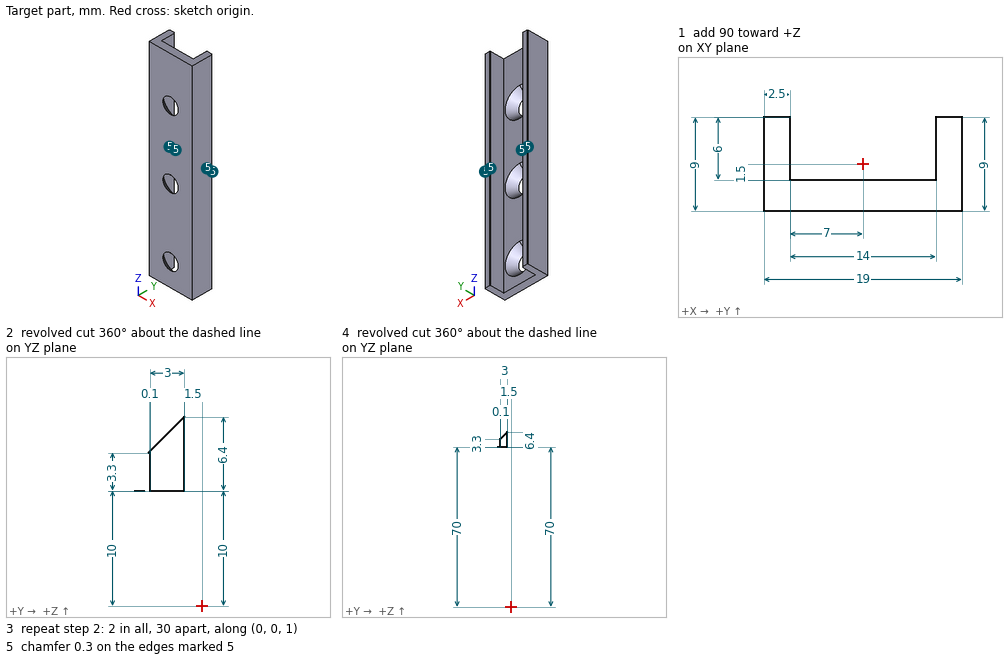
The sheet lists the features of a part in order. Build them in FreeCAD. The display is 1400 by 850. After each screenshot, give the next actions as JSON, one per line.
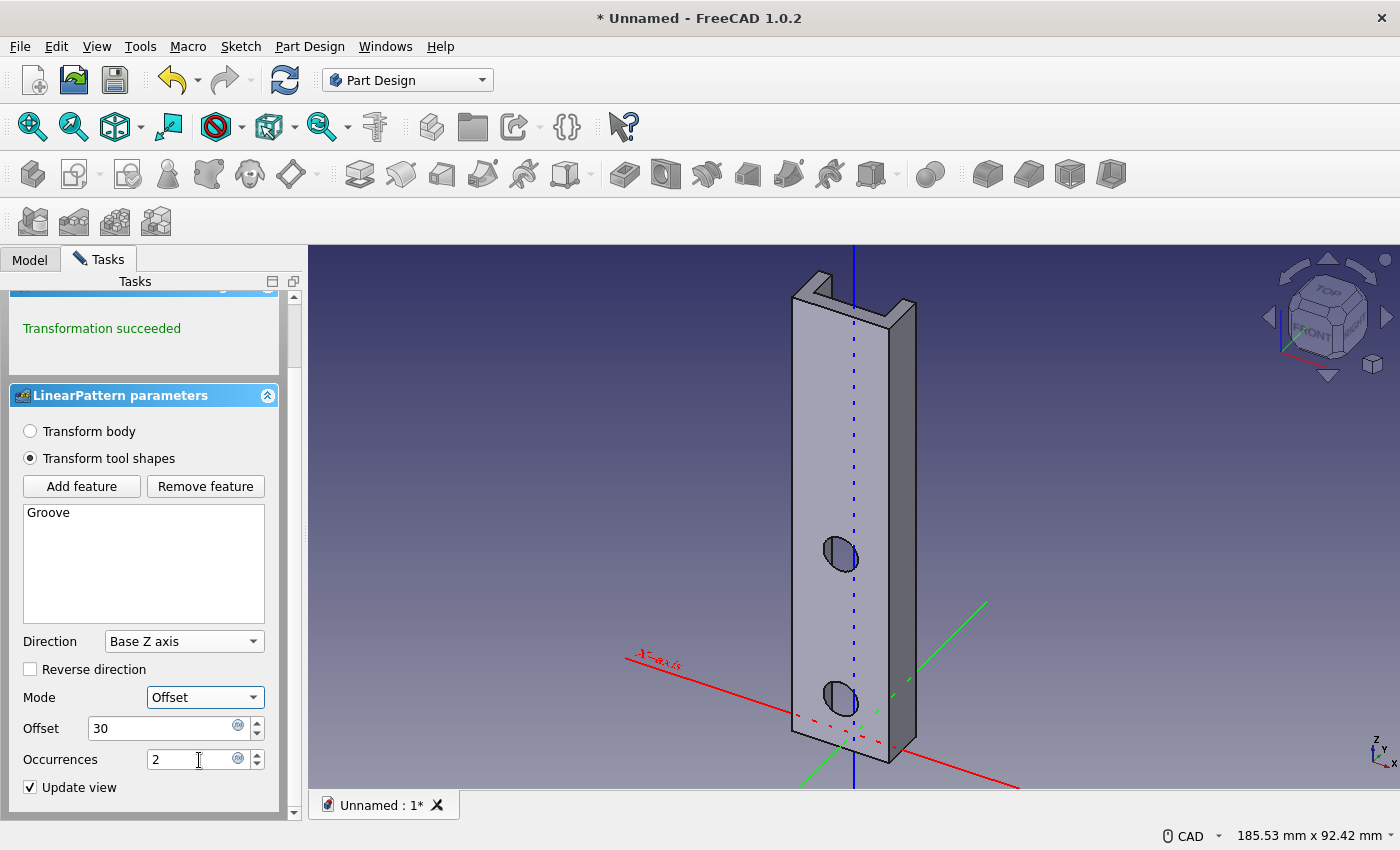
{"action": "scroll", "coordinate": [294, 556], "scroll_direction": "up", "scroll_amount": 3}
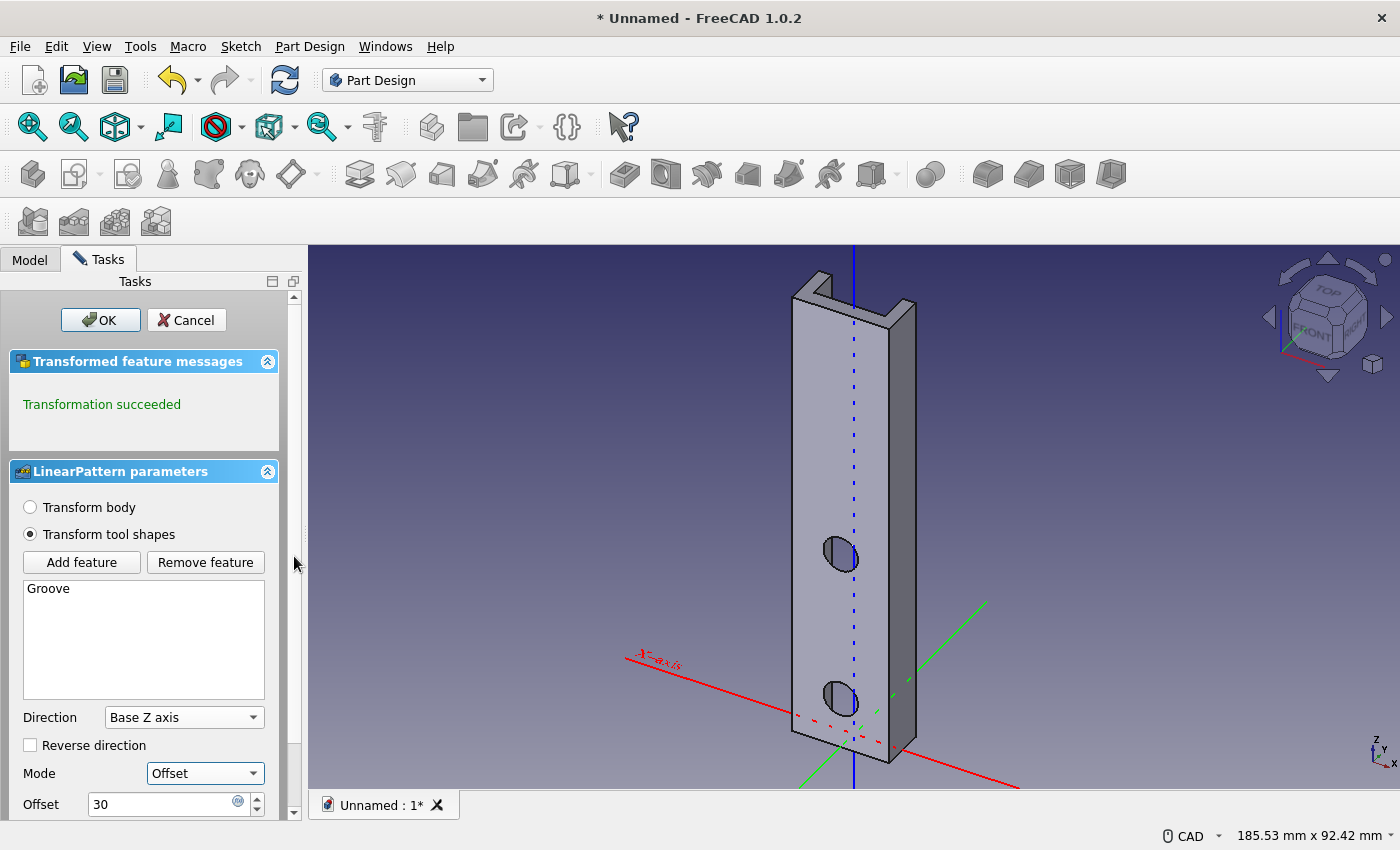
{"action": "left_click", "coordinate": [101, 320]}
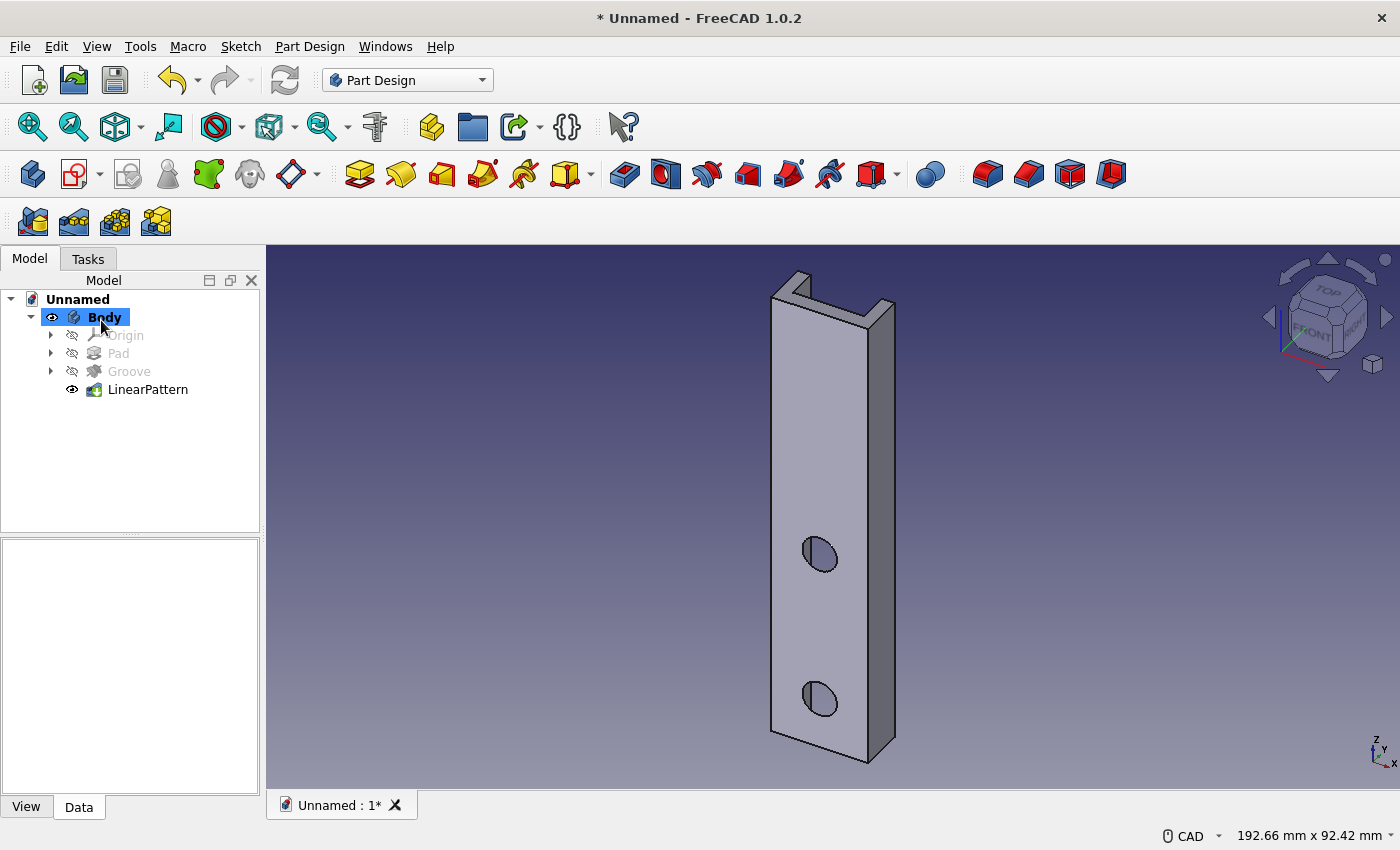
{"action": "left_click", "coordinate": [74, 174]}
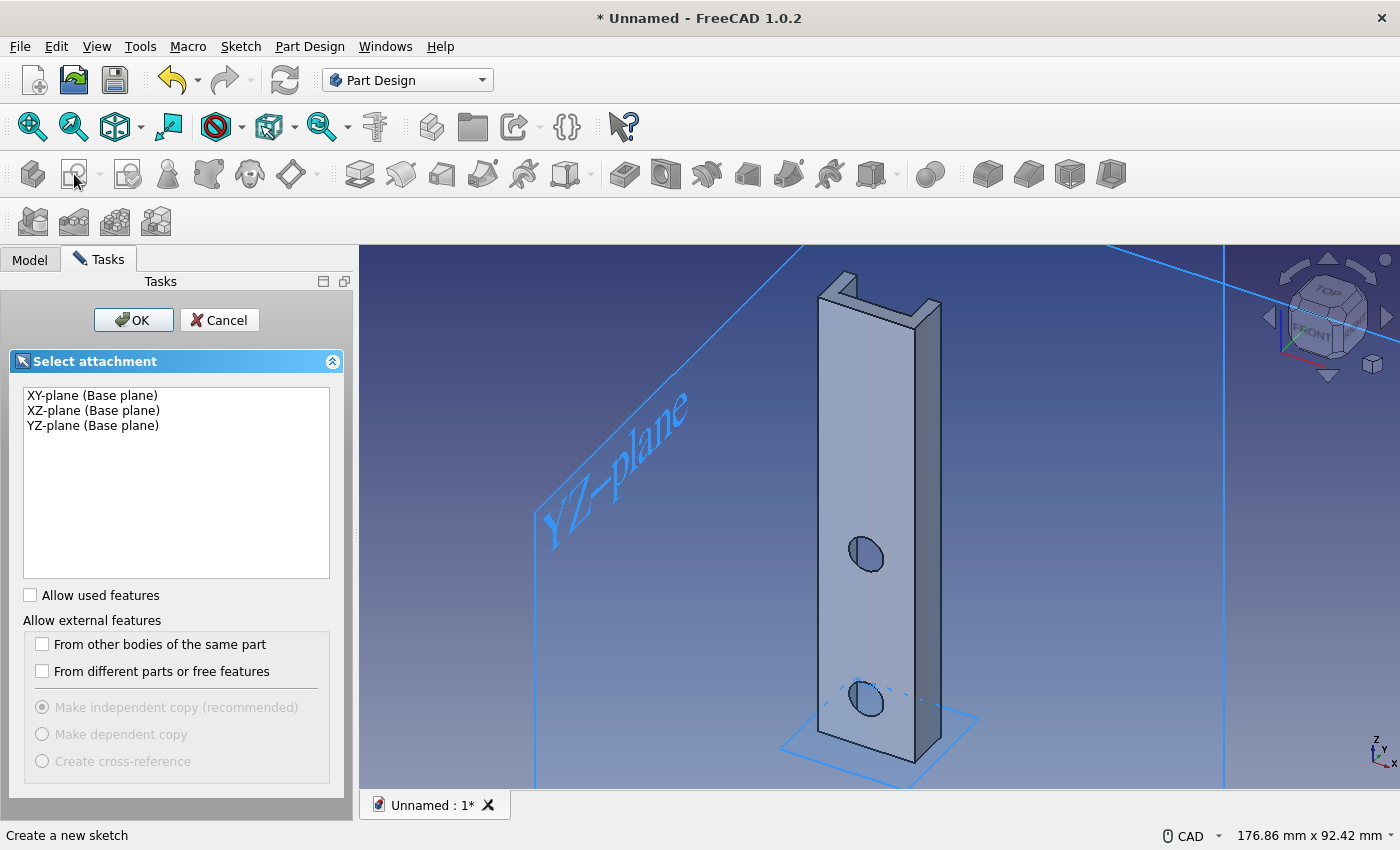
{"action": "left_click", "coordinate": [84, 426]}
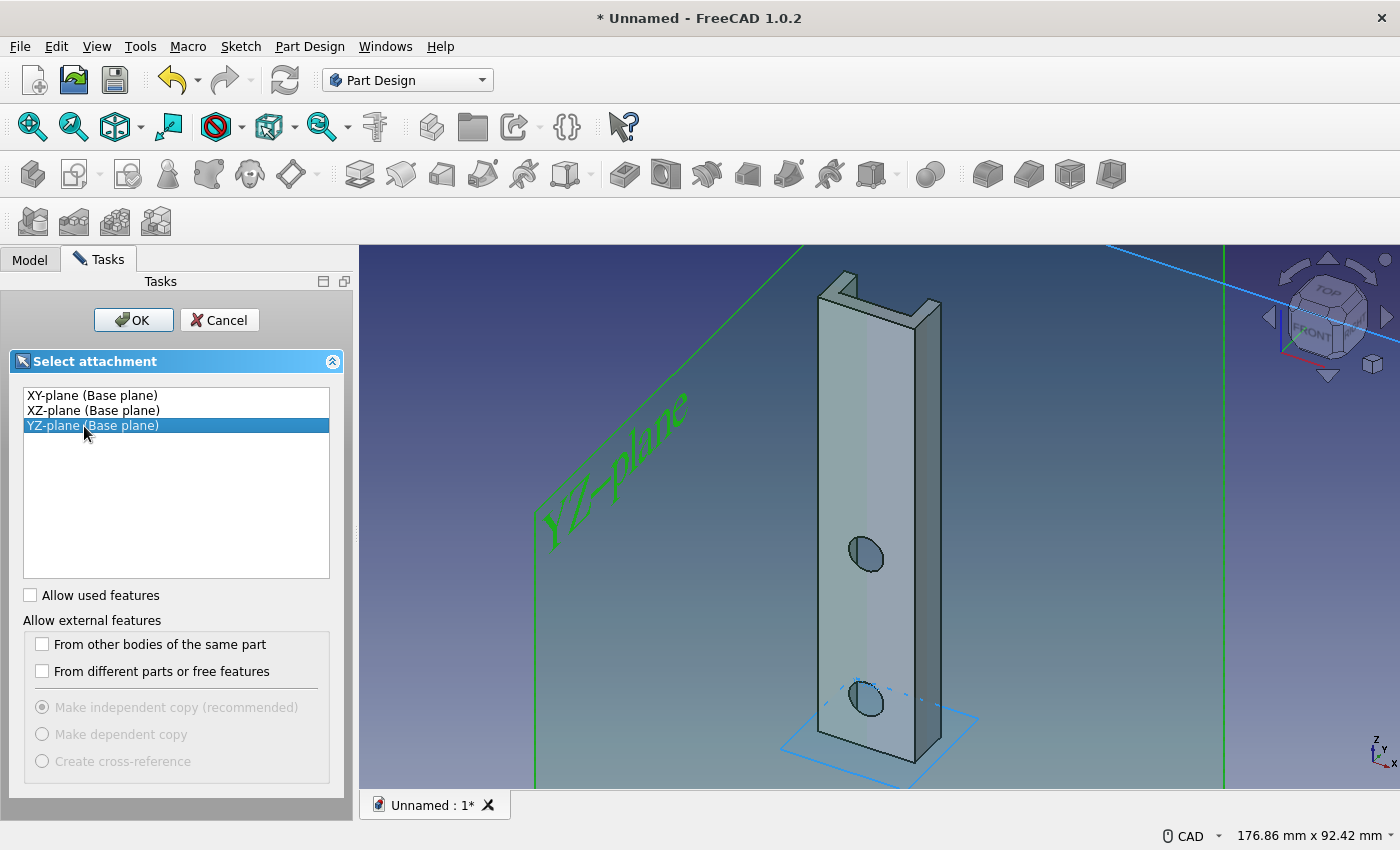
{"action": "left_click", "coordinate": [134, 320]}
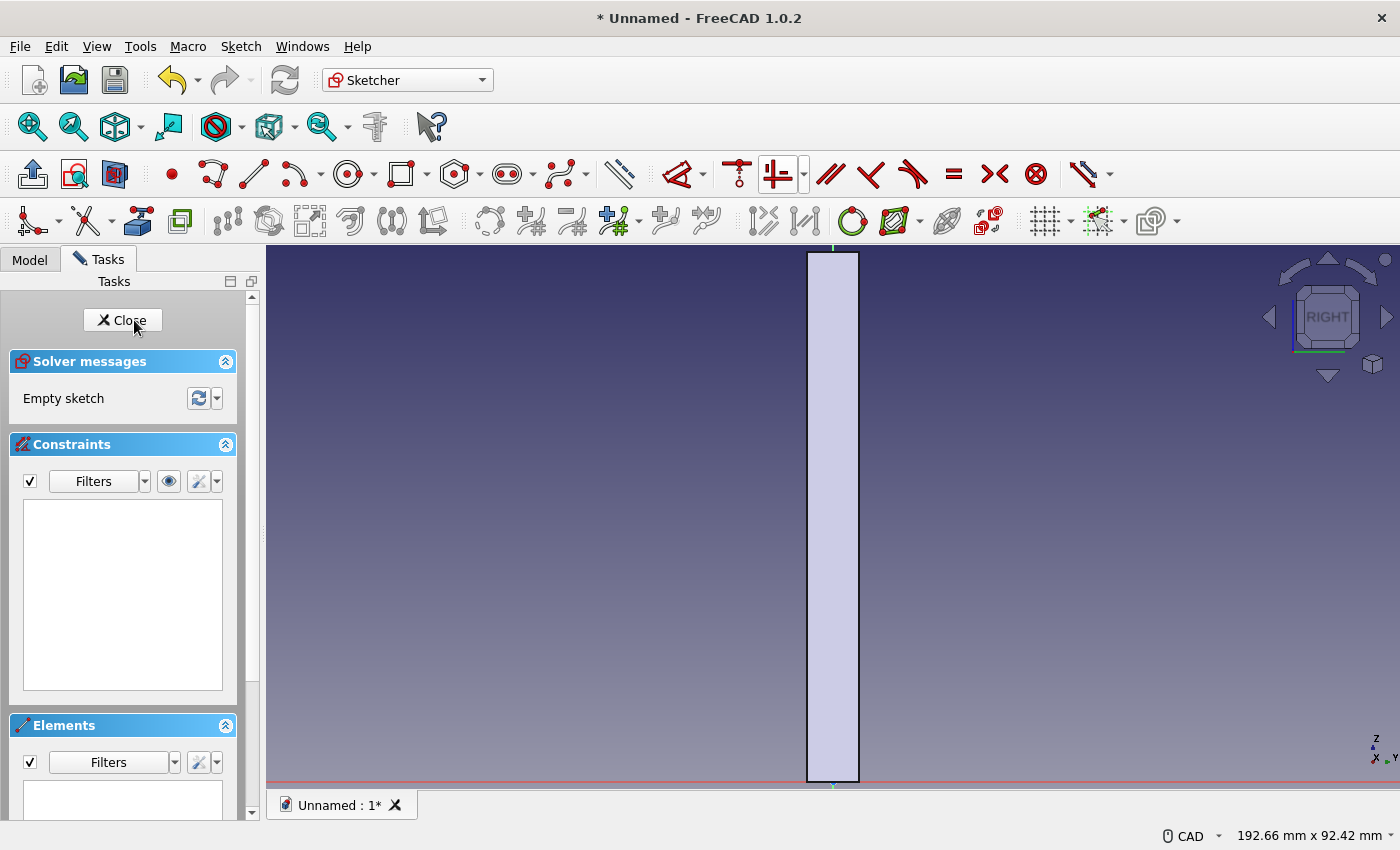
{"action": "left_click", "coordinate": [115, 174]}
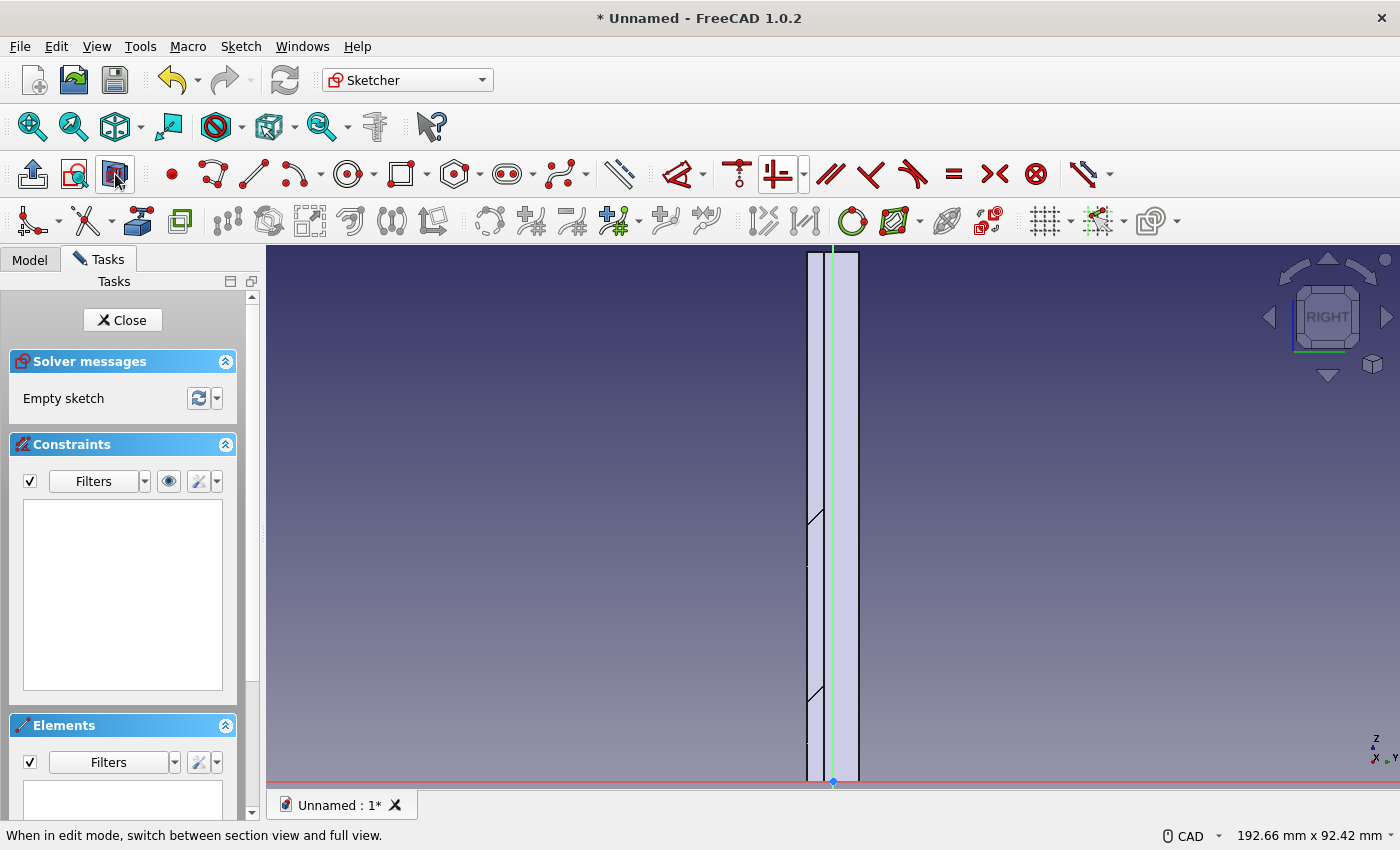
{"action": "scroll", "coordinate": [817, 330], "scroll_direction": "up", "scroll_amount": 11}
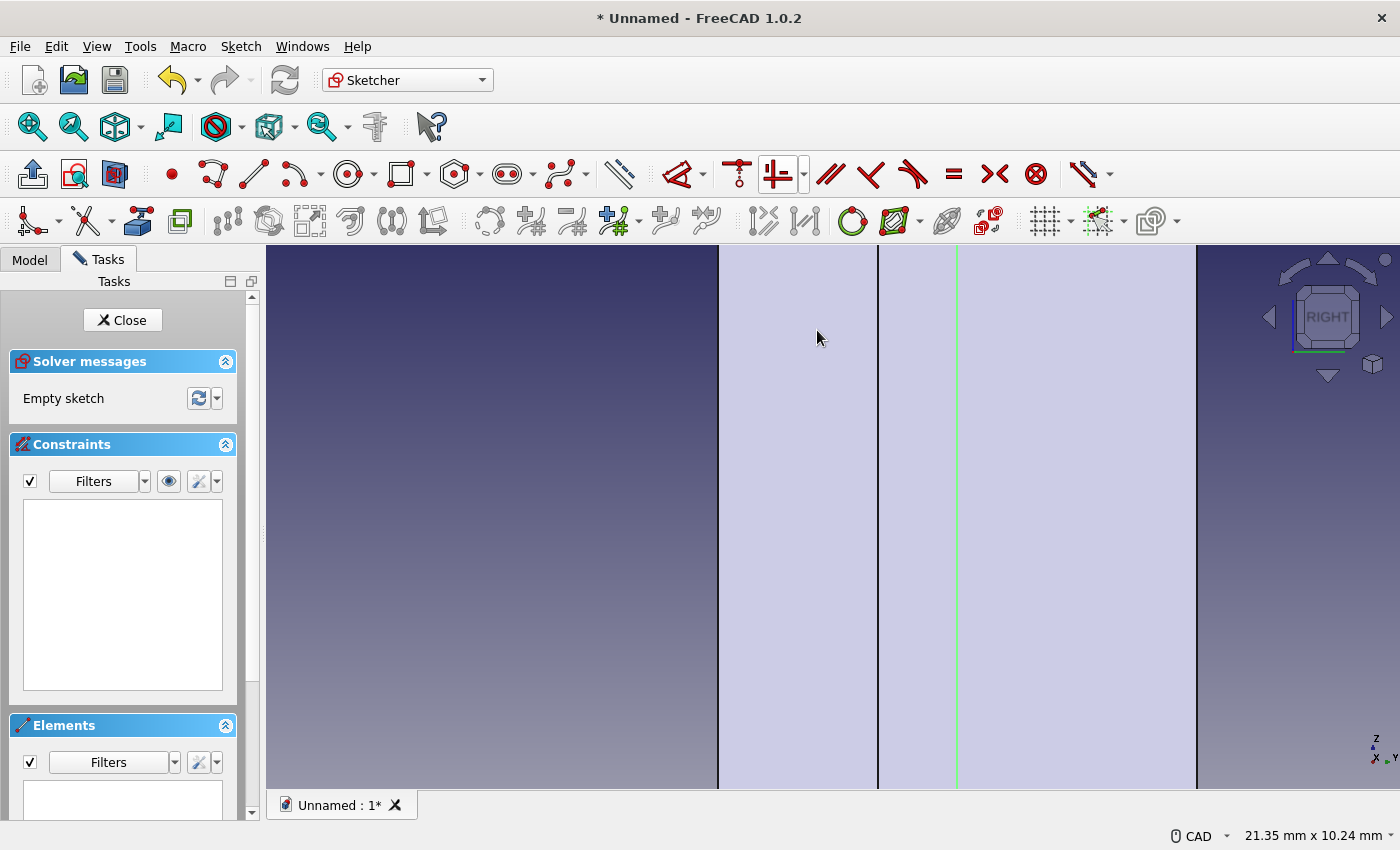
{"action": "key", "text": "g m"}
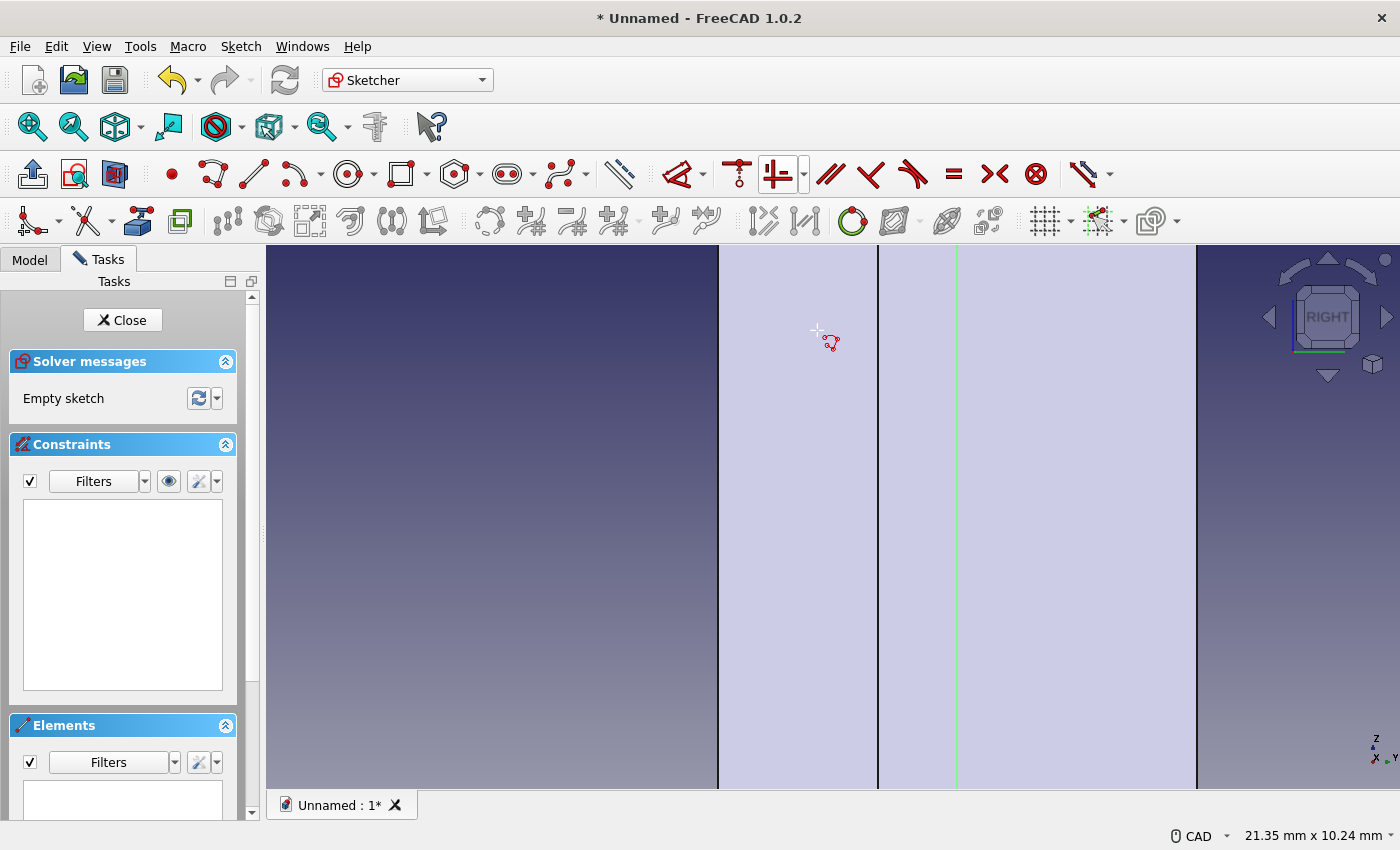
{"action": "left_click", "coordinate": [878, 688]}
{"action": "left_click", "coordinate": [878, 348]}
{"action": "left_click", "coordinate": [713, 513]}